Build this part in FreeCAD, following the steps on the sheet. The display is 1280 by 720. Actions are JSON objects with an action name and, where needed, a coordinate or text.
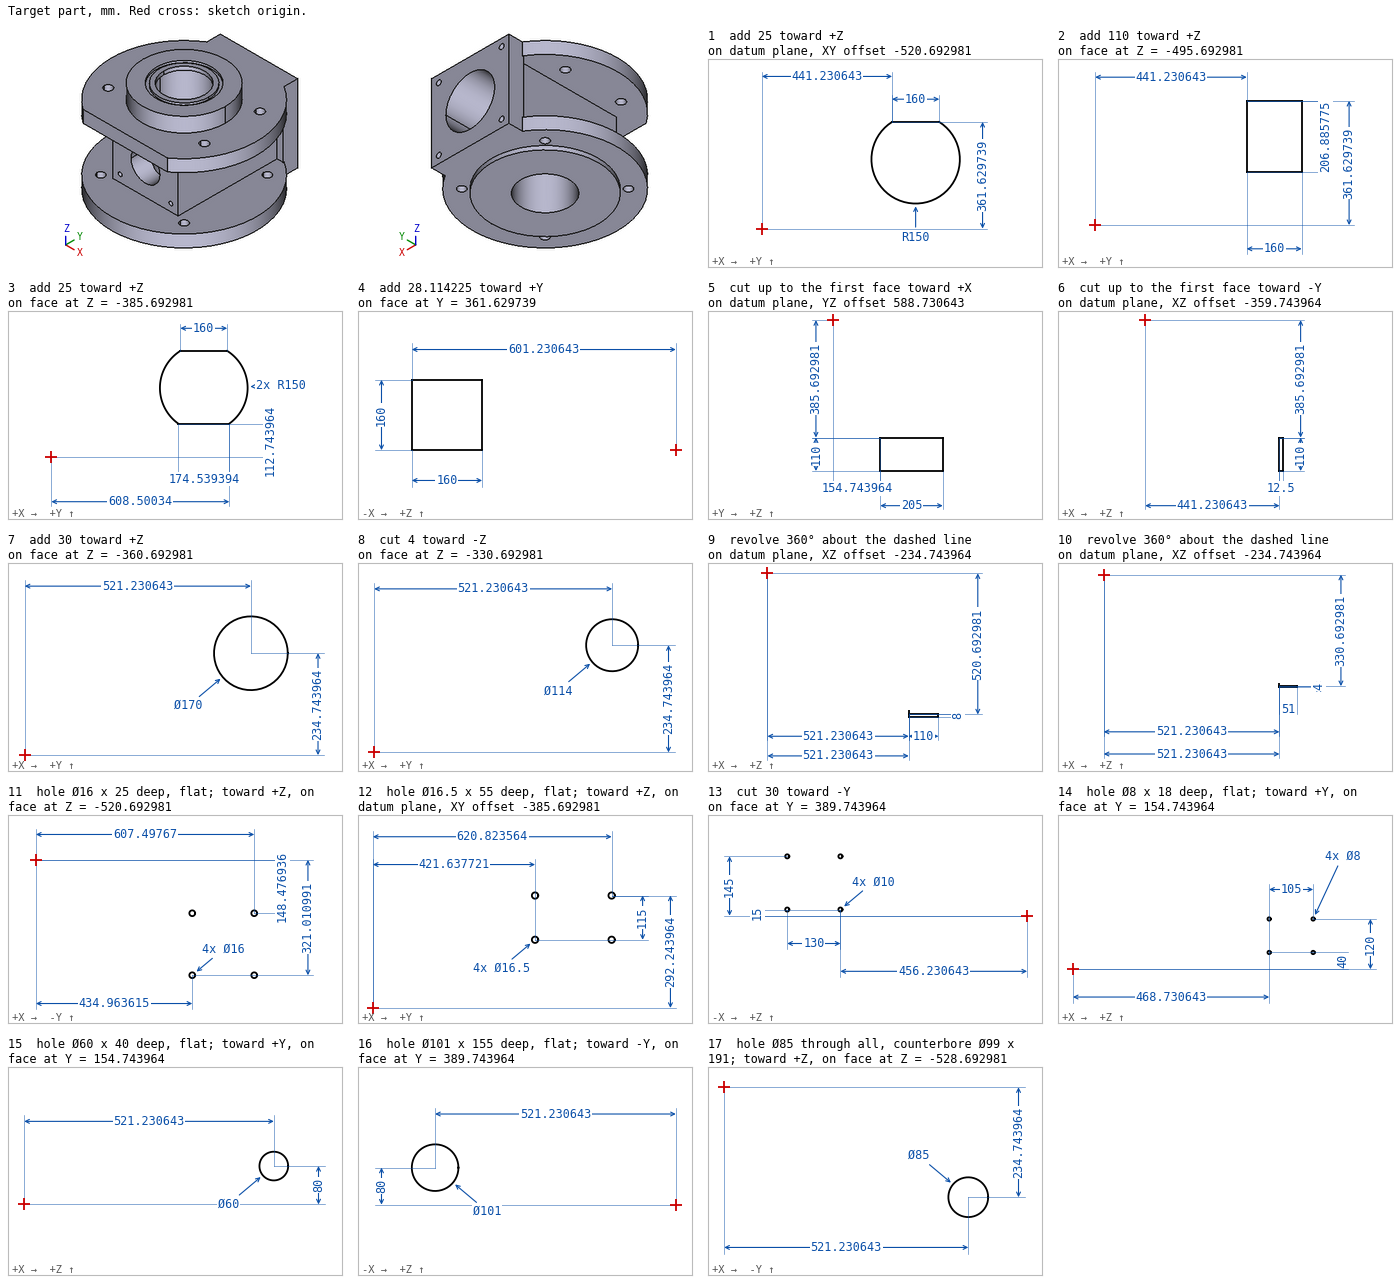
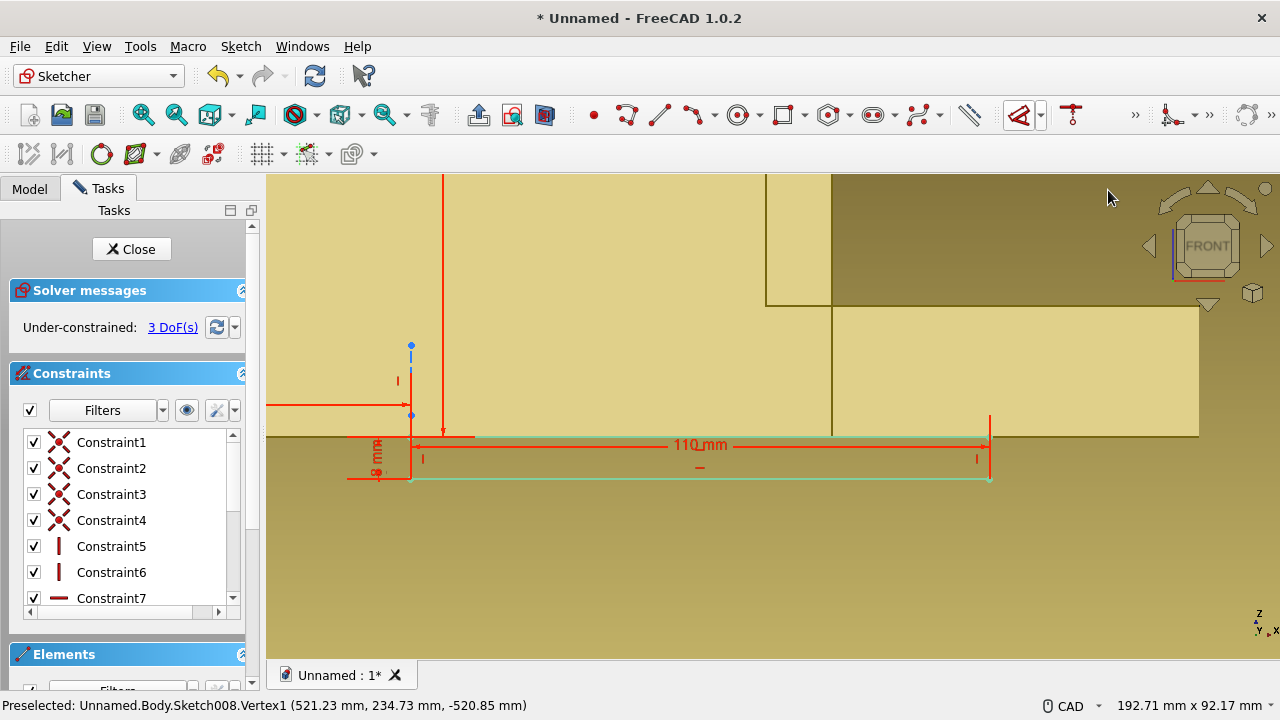
{"action": "left_click", "coordinate": [411, 415]}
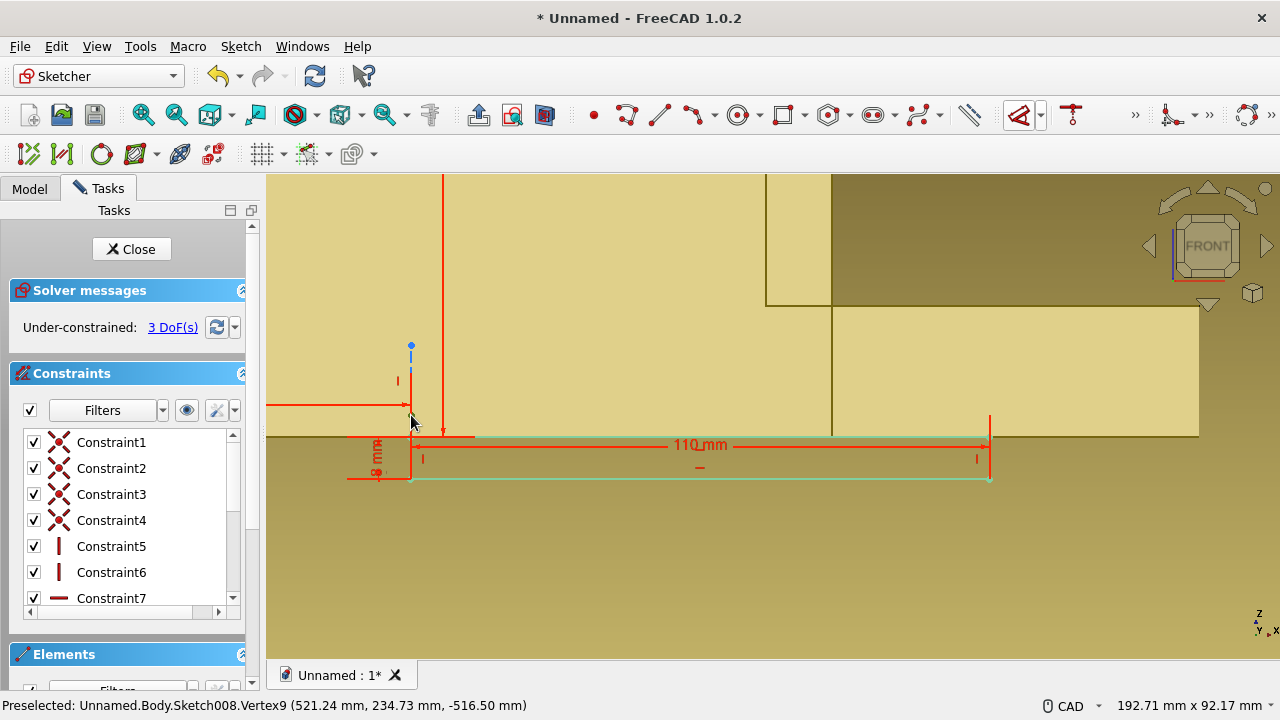
{"action": "key", "text": "l"}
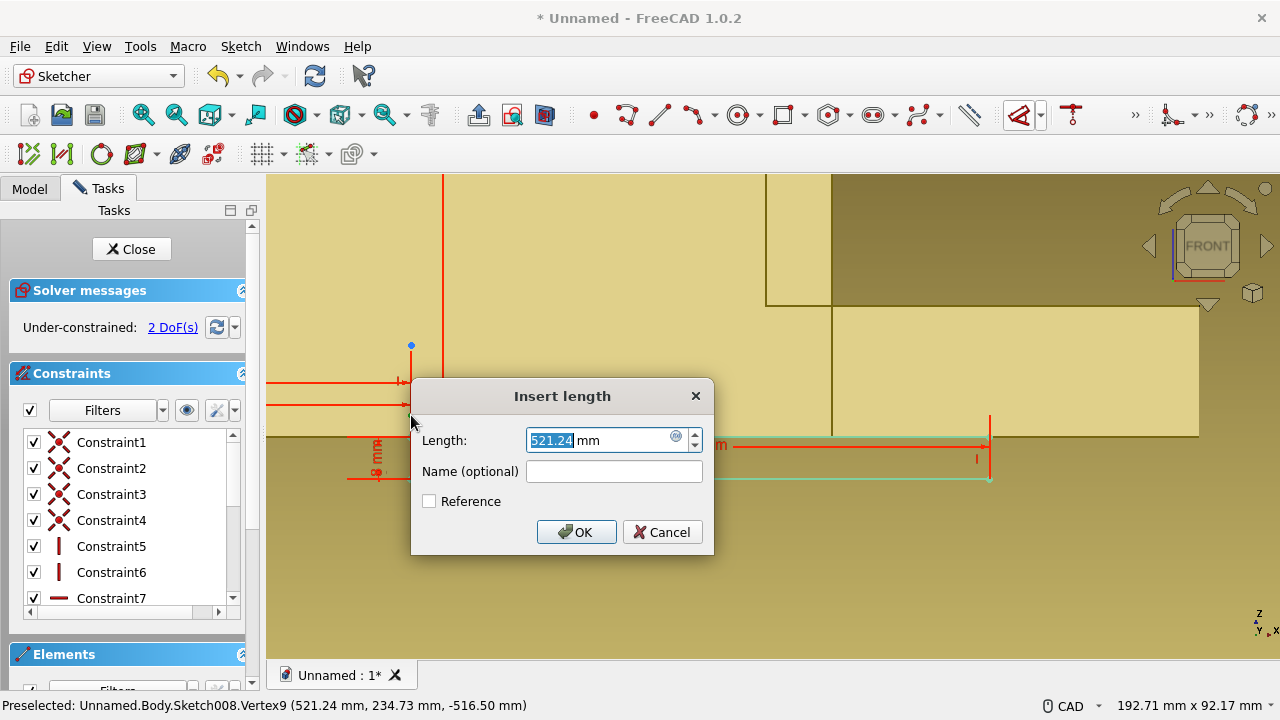
{"action": "type", "text": "521.230643"}
{"action": "key", "text": "Return"}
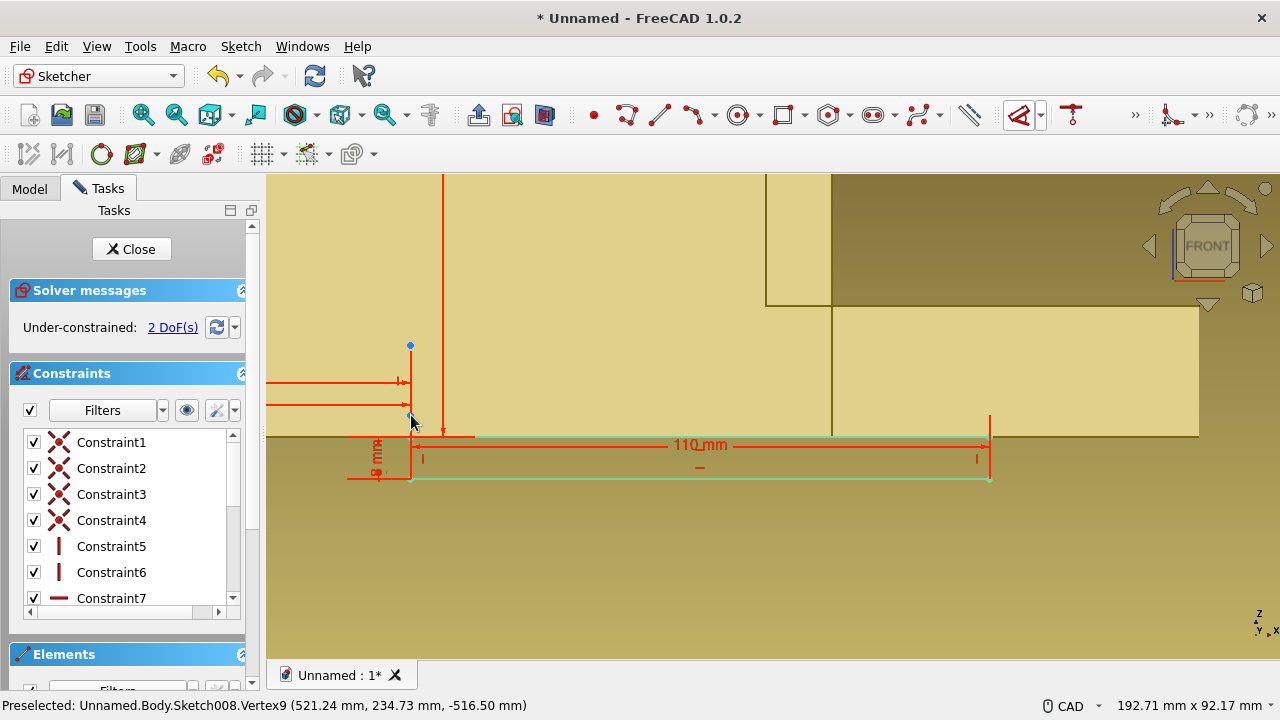
{"action": "left_click", "coordinate": [132, 249]}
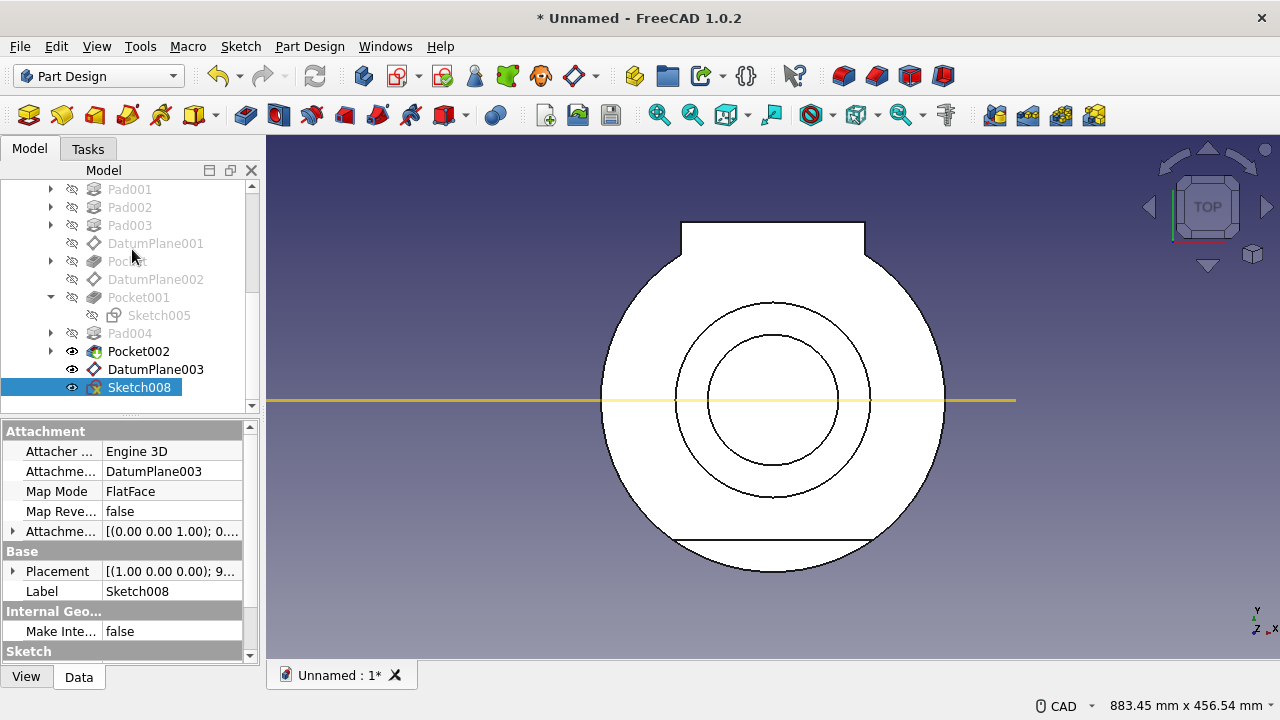
{"action": "left_click", "coordinate": [62, 116]}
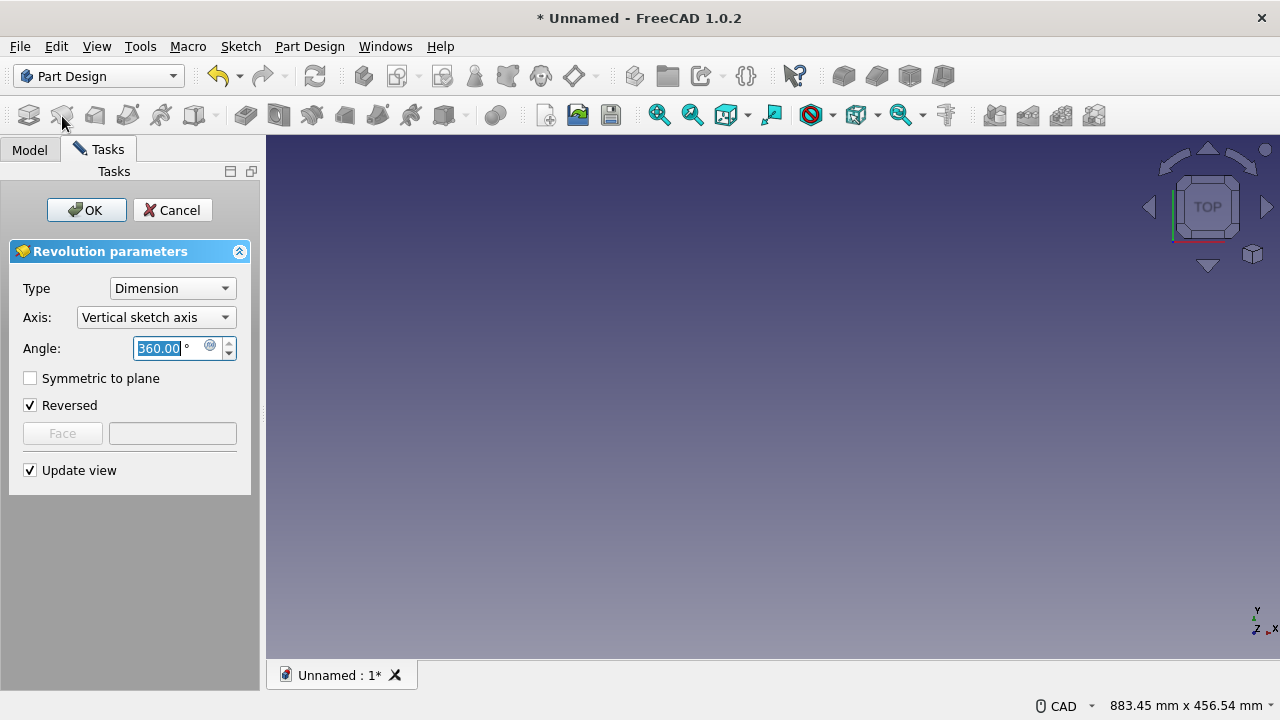
{"action": "left_click", "coordinate": [157, 318]}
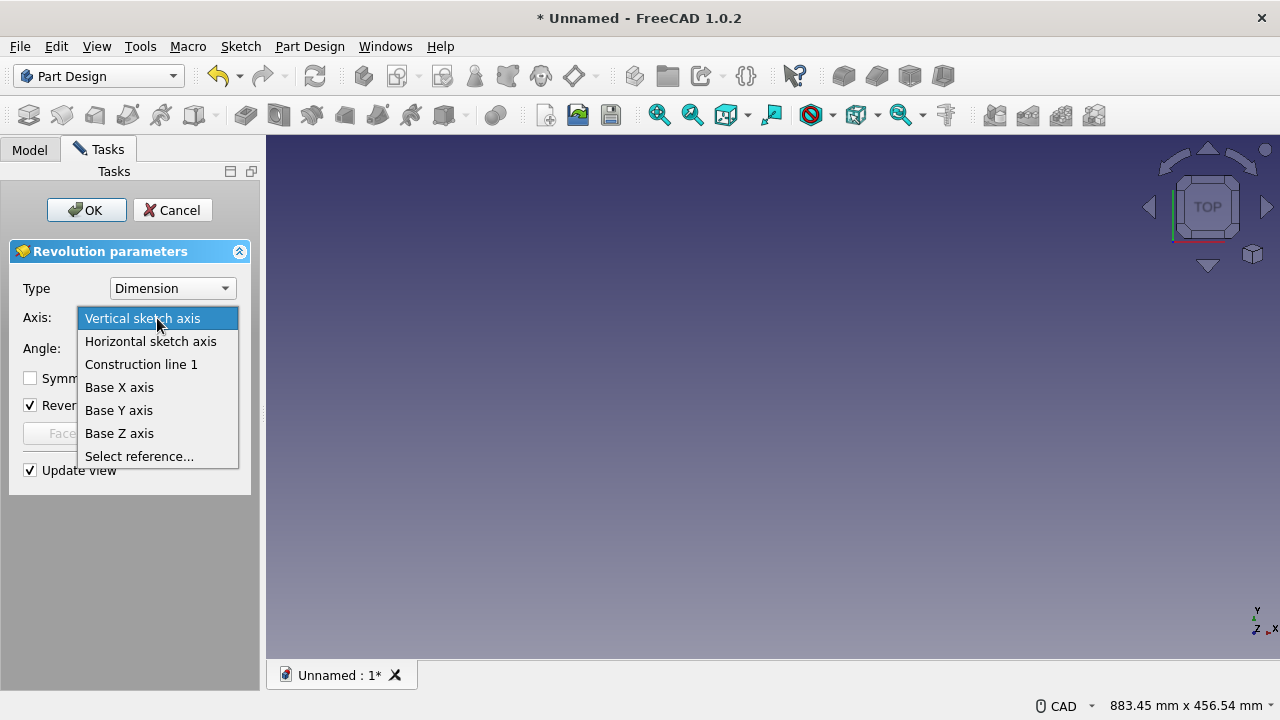
{"action": "left_click", "coordinate": [156, 364]}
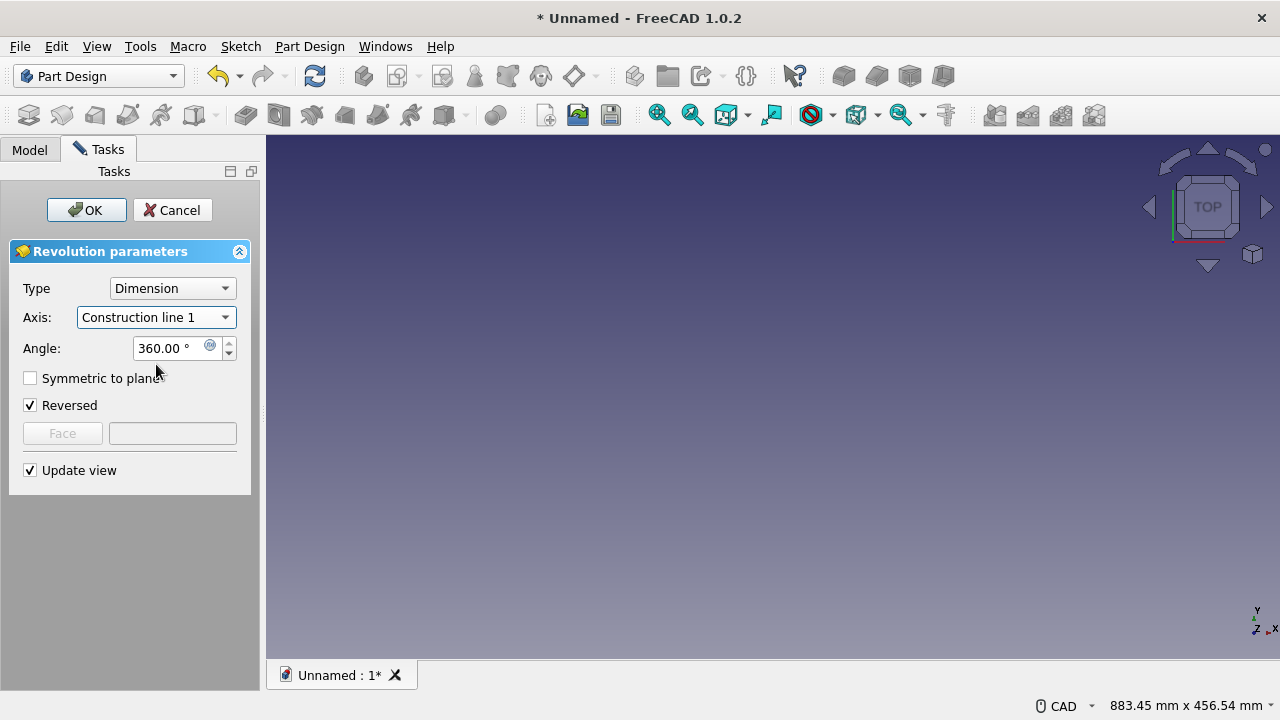
{"action": "left_click", "coordinate": [87, 210]}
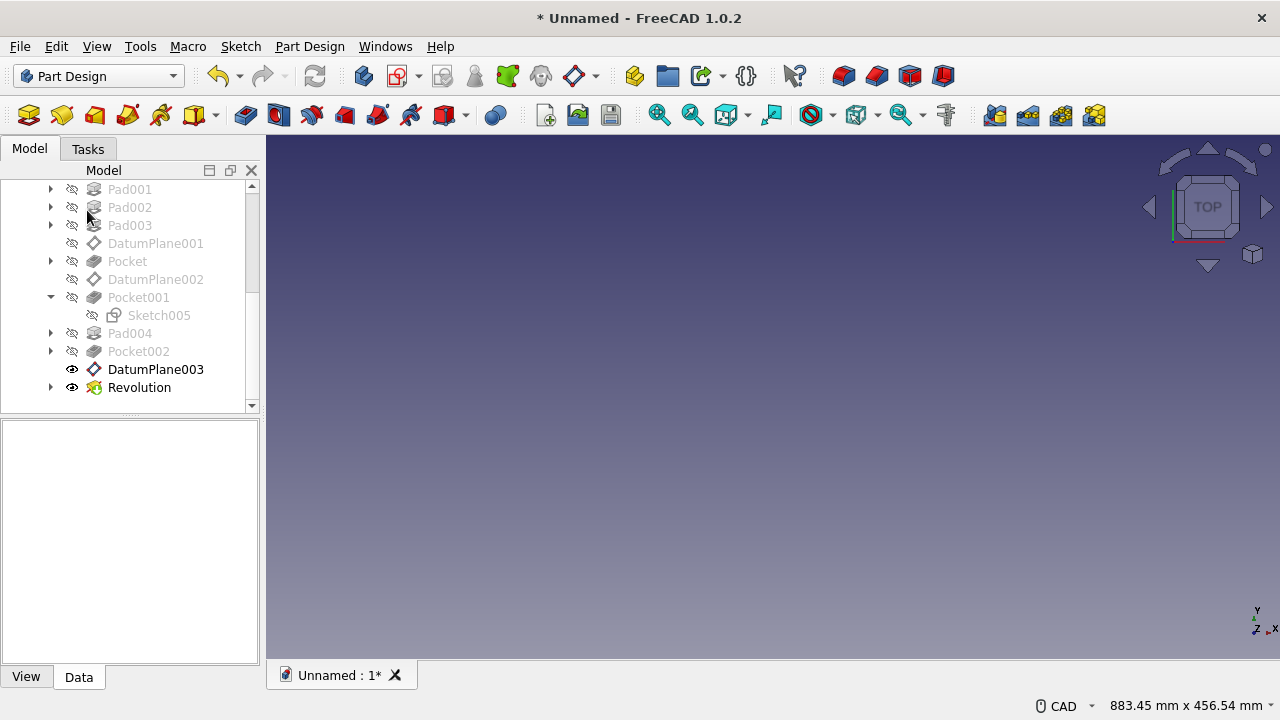
{"action": "left_click", "coordinate": [117, 369]}
{"action": "key", "text": "space"}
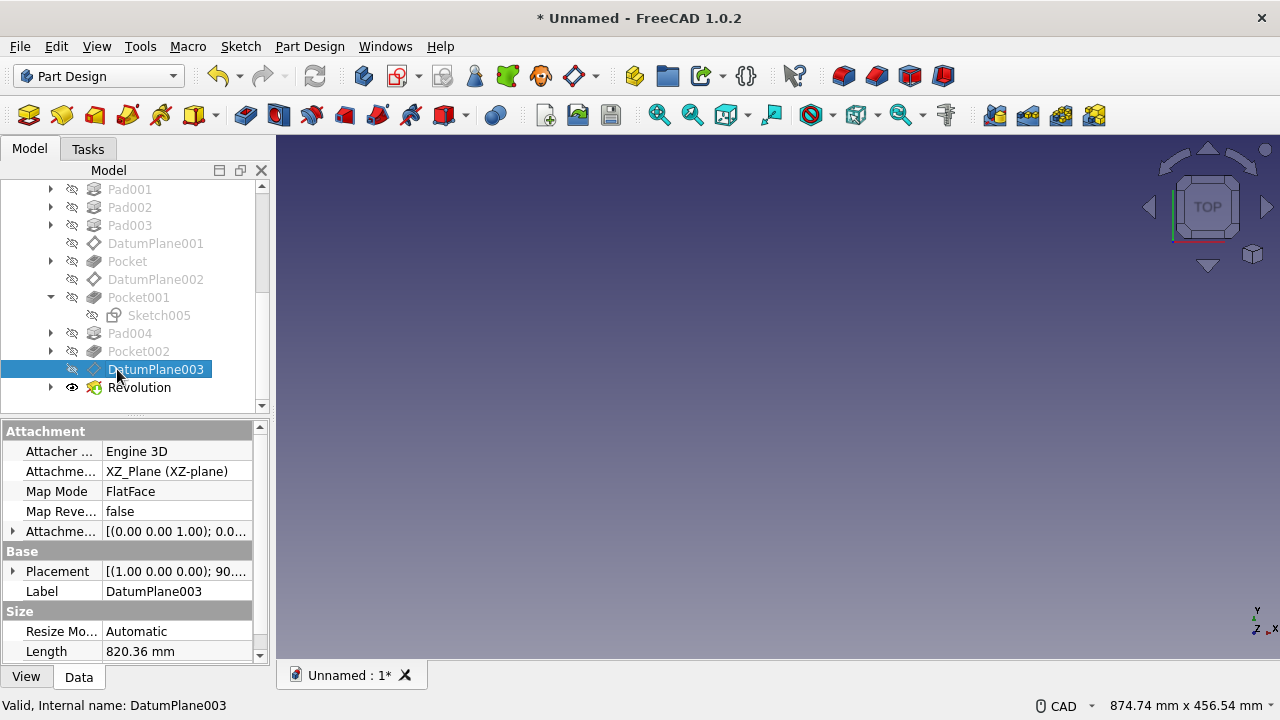
{"action": "left_click", "coordinate": [660, 116]}